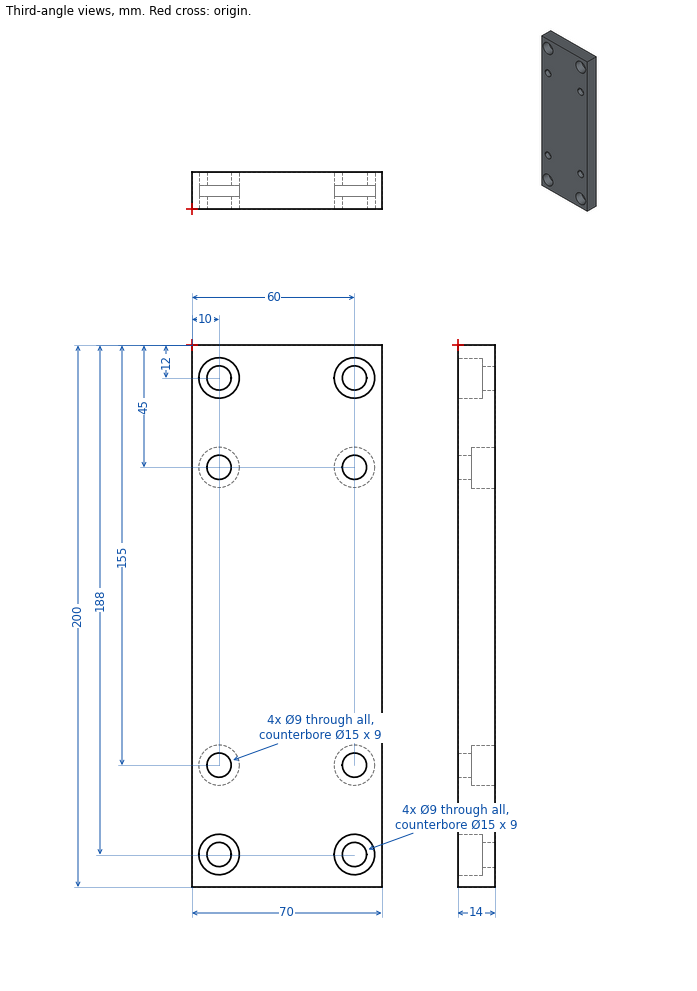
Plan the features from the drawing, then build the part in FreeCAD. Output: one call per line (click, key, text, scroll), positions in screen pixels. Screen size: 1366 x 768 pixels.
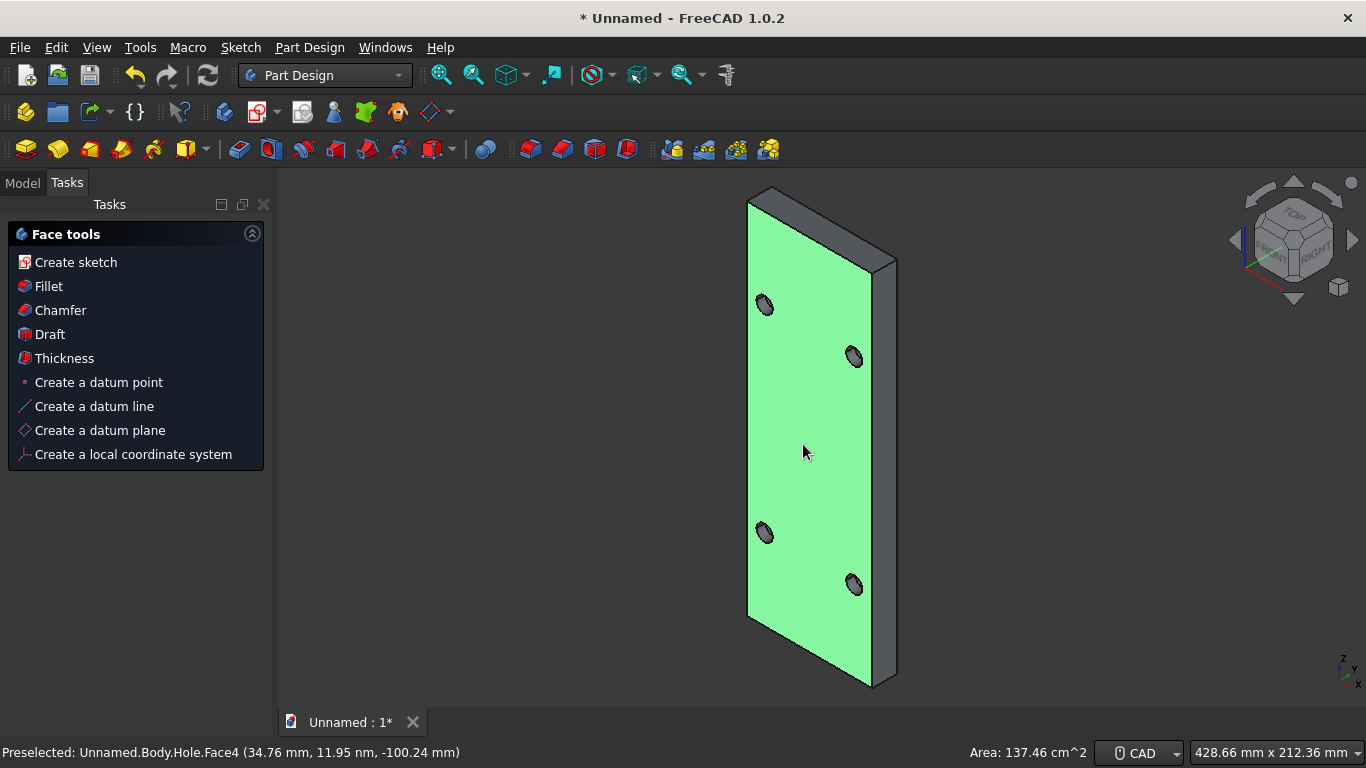
click(258, 112)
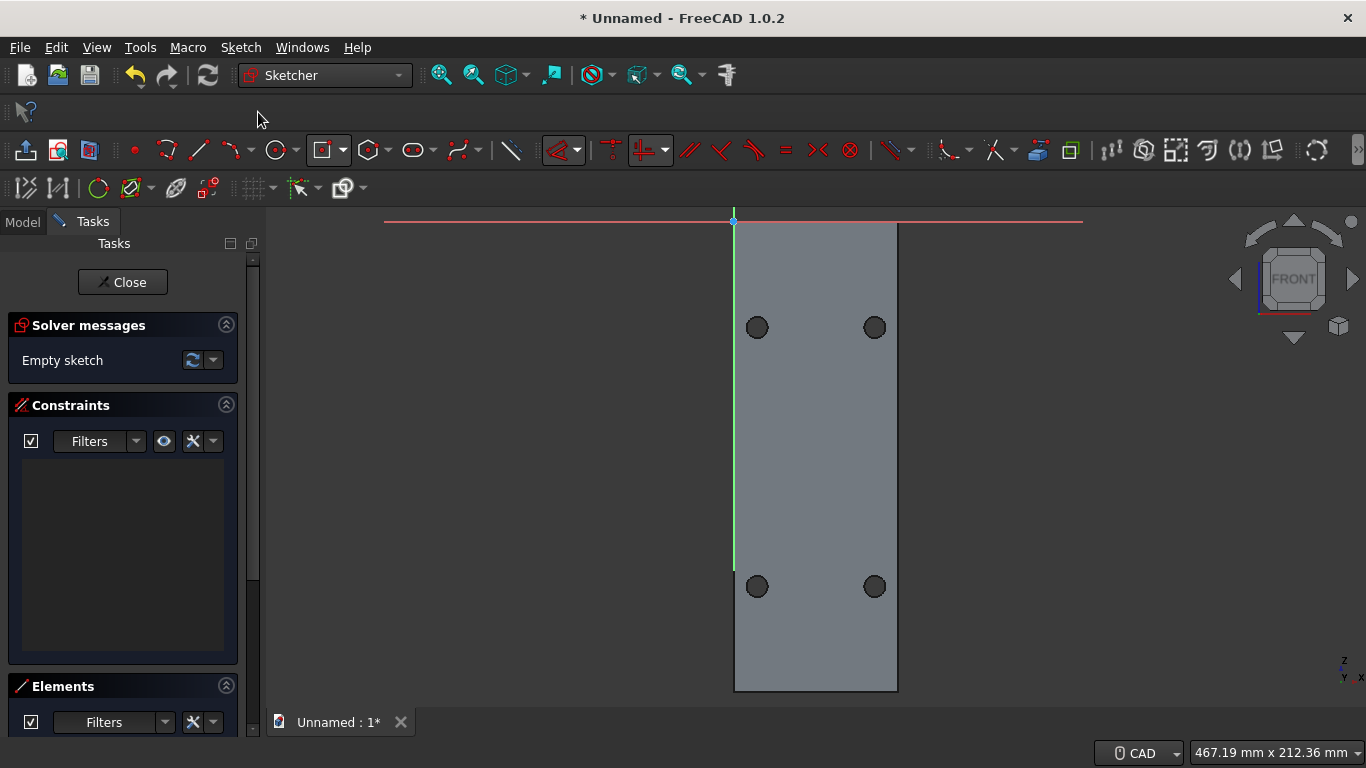
scroll(621, 475, down, 2)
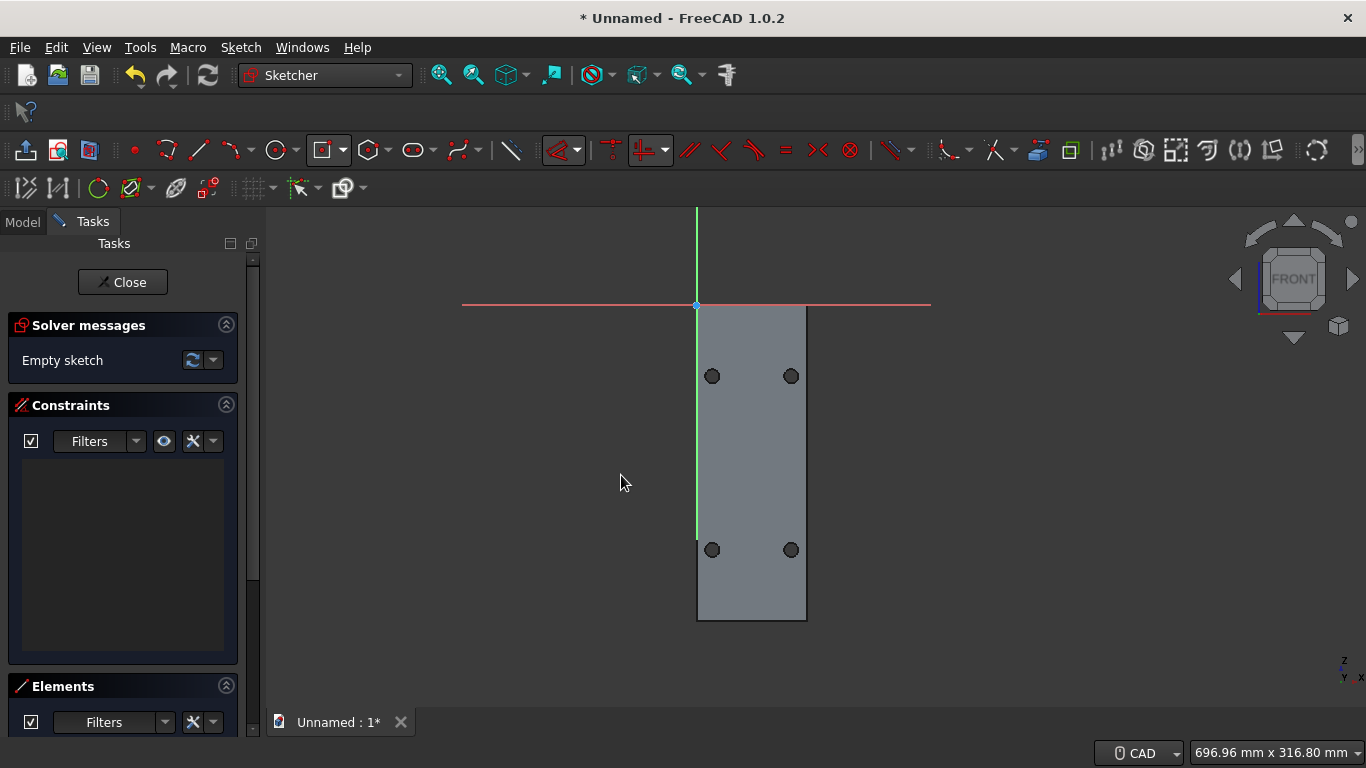
key(g)
key(c)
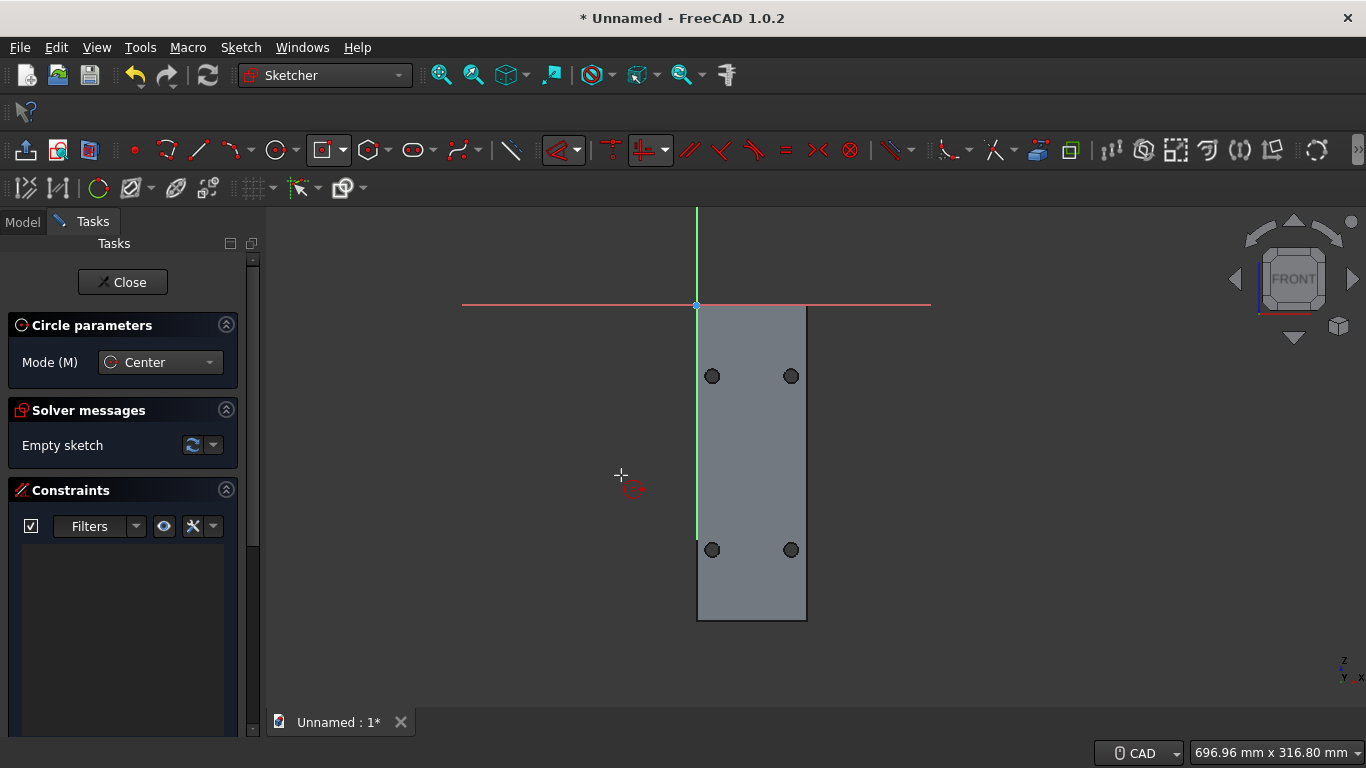
scroll(791, 602, up, 6)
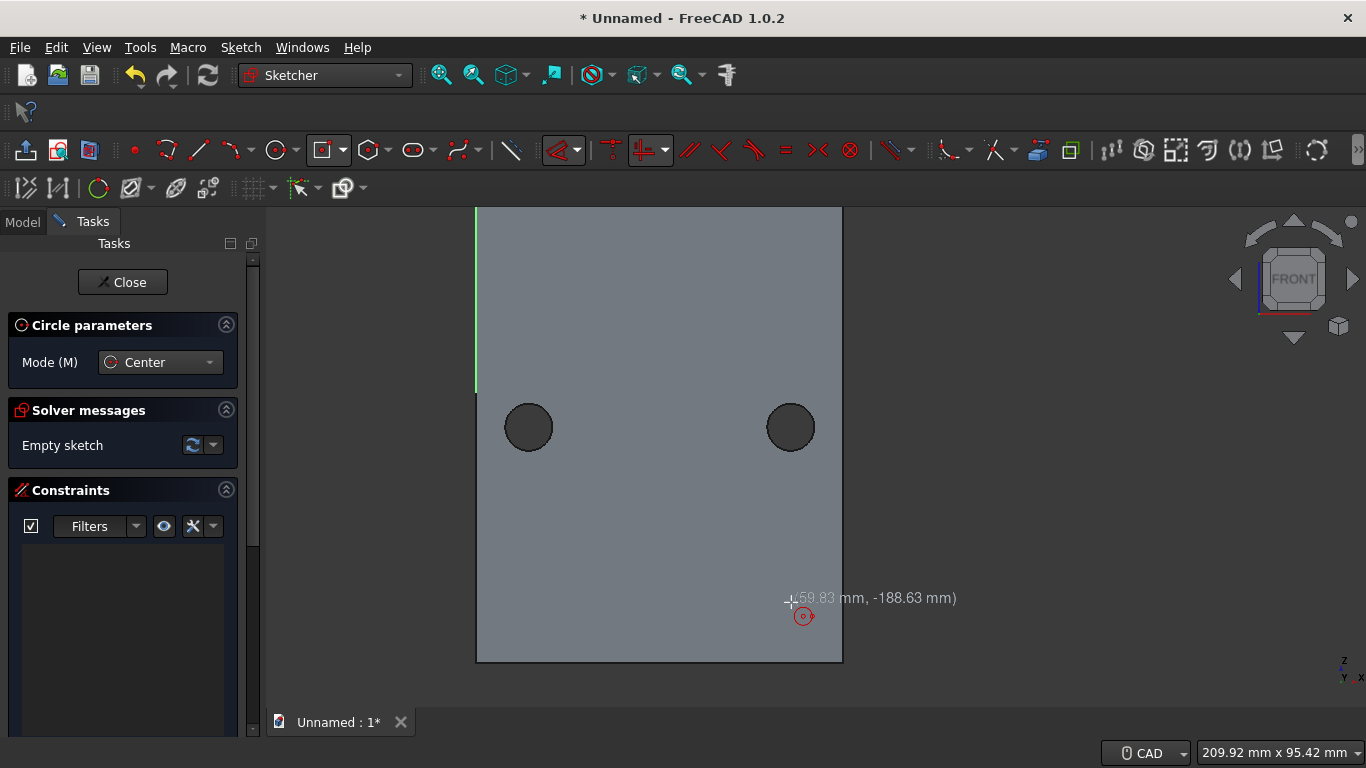
click(791, 600)
click(807, 583)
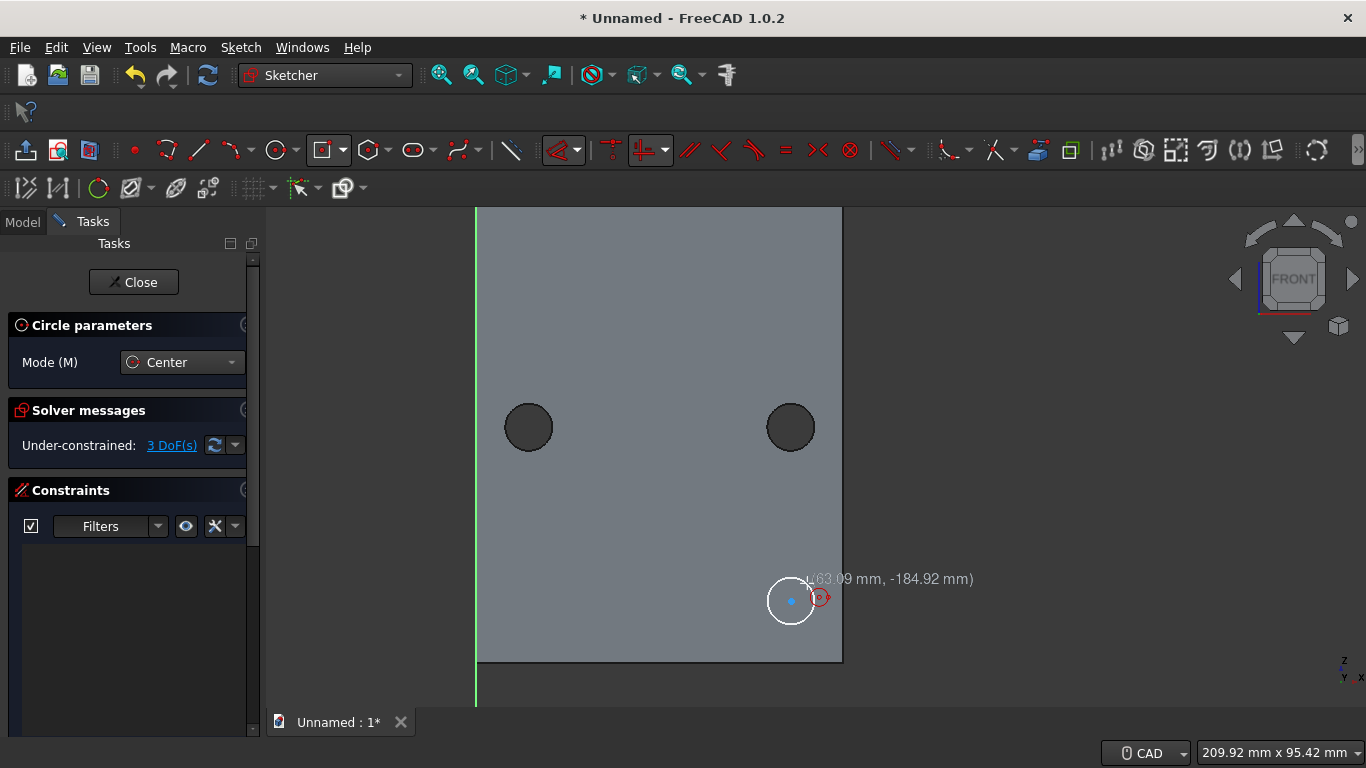
click(529, 600)
click(545, 583)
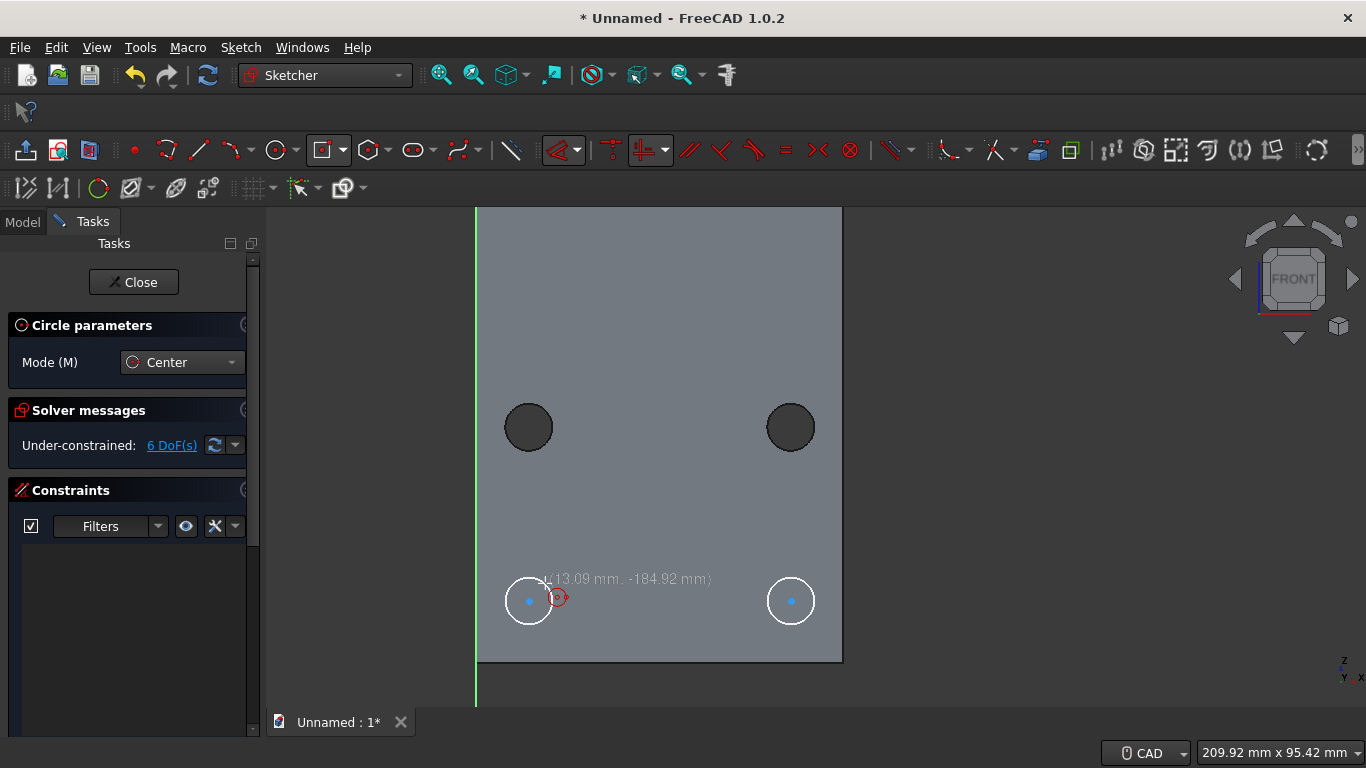
scroll(792, 603, down, 6)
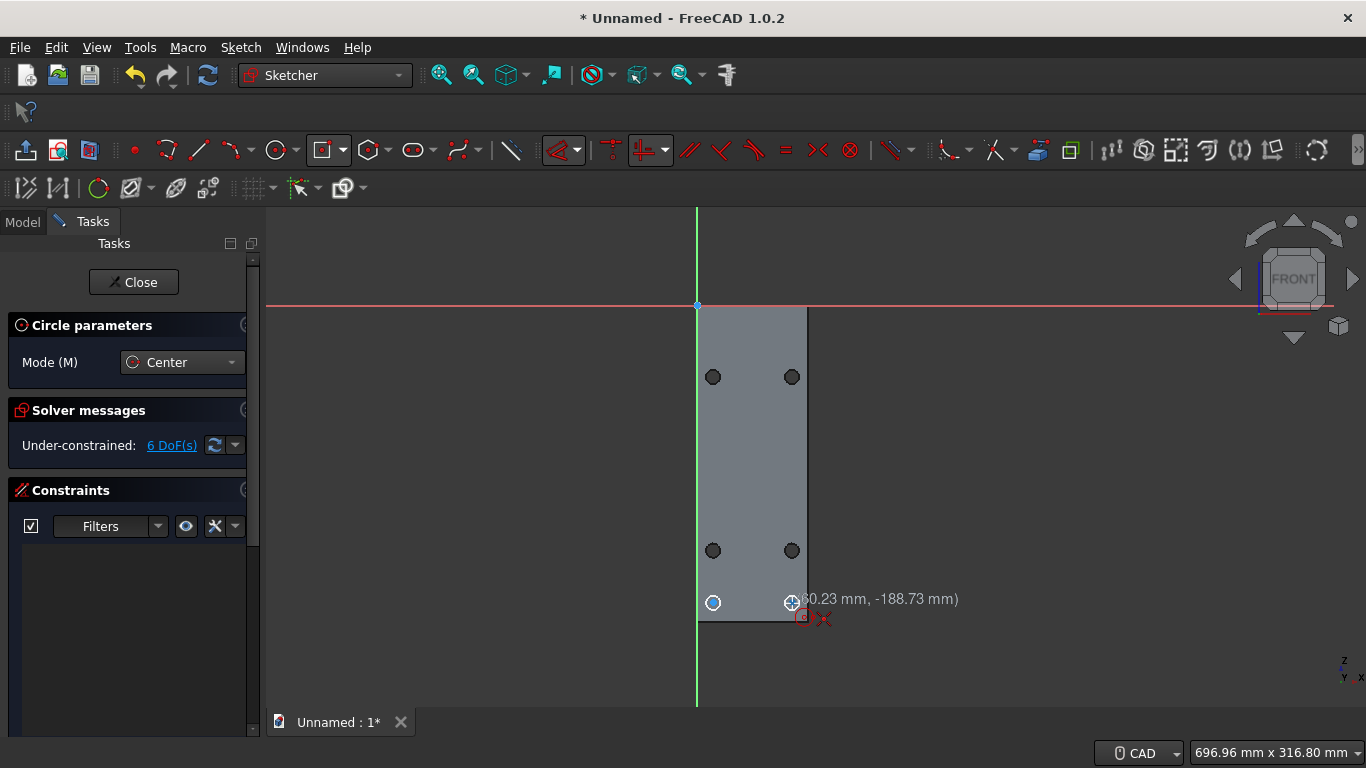
scroll(713, 325, up, 6)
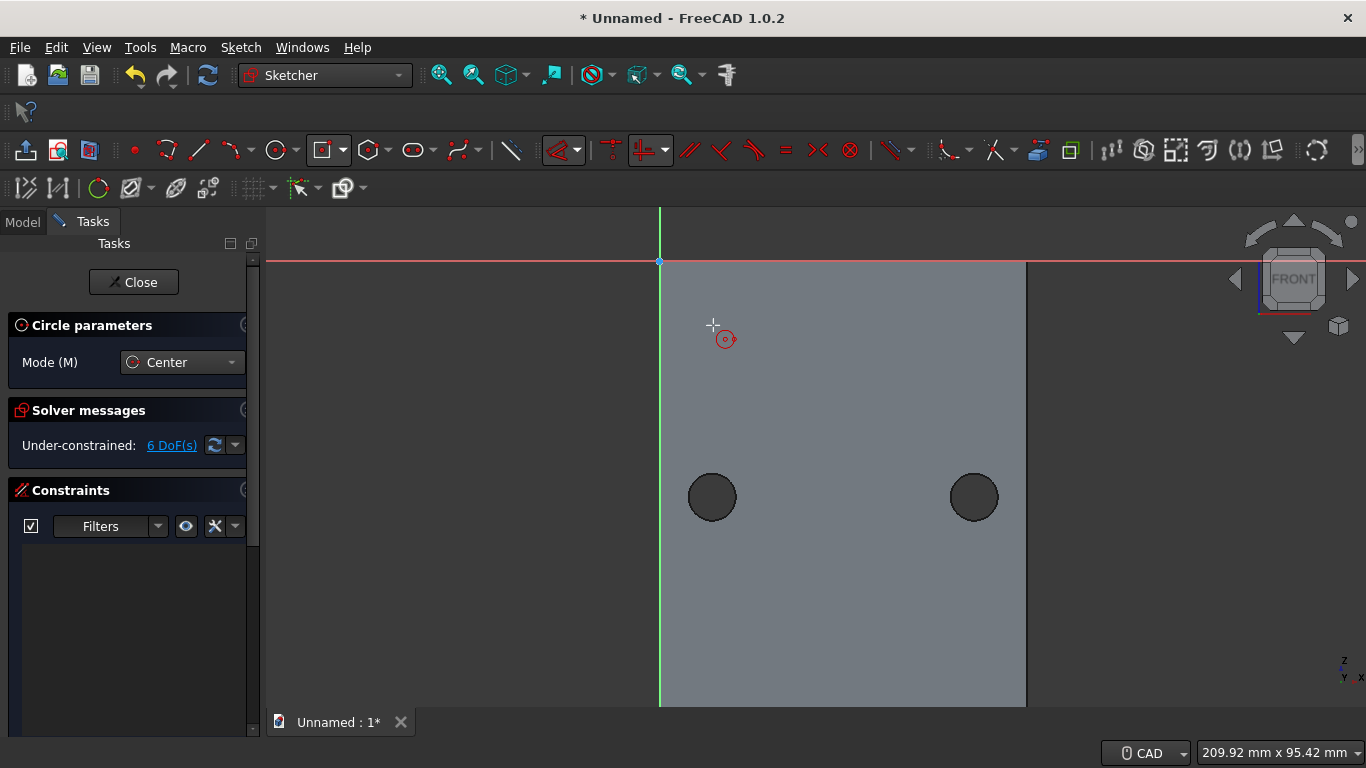
click(712, 324)
click(729, 308)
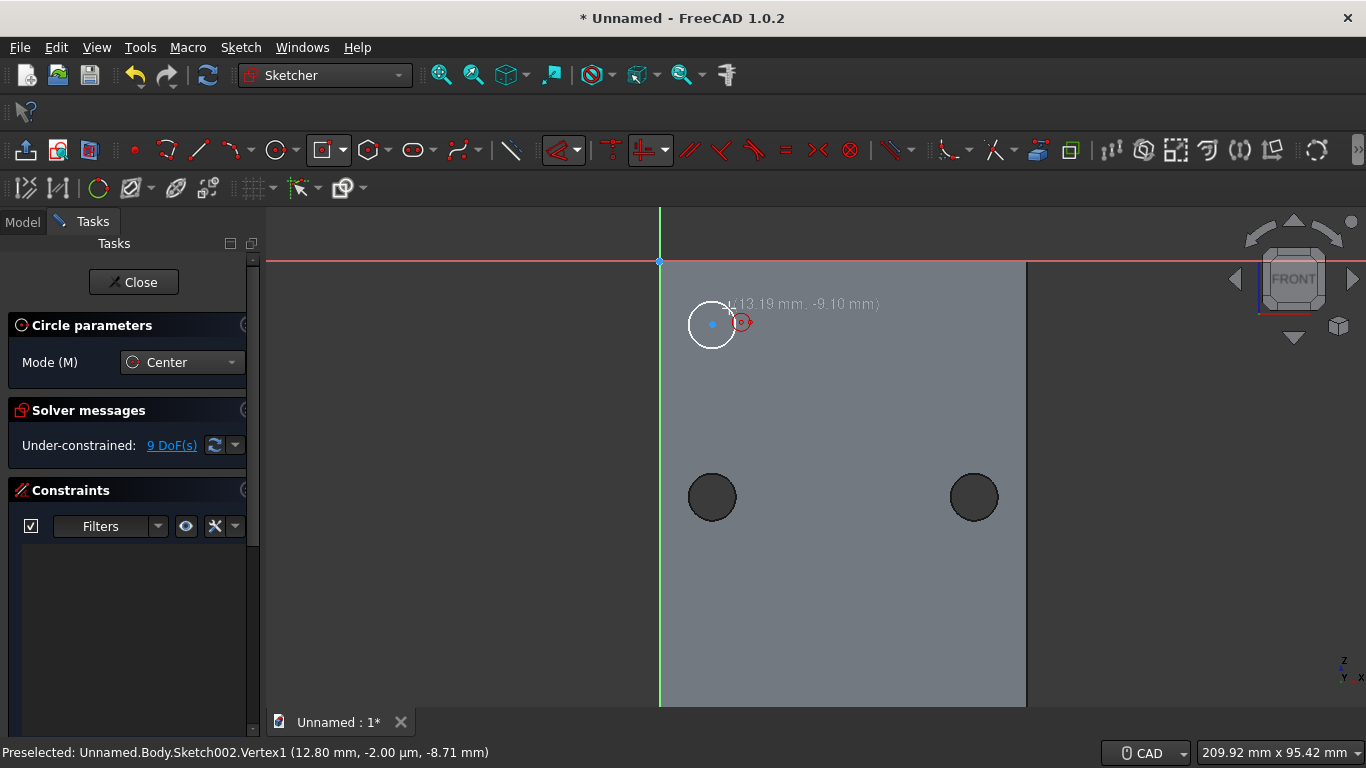
click(974, 324)
click(991, 308)
key(Escape)